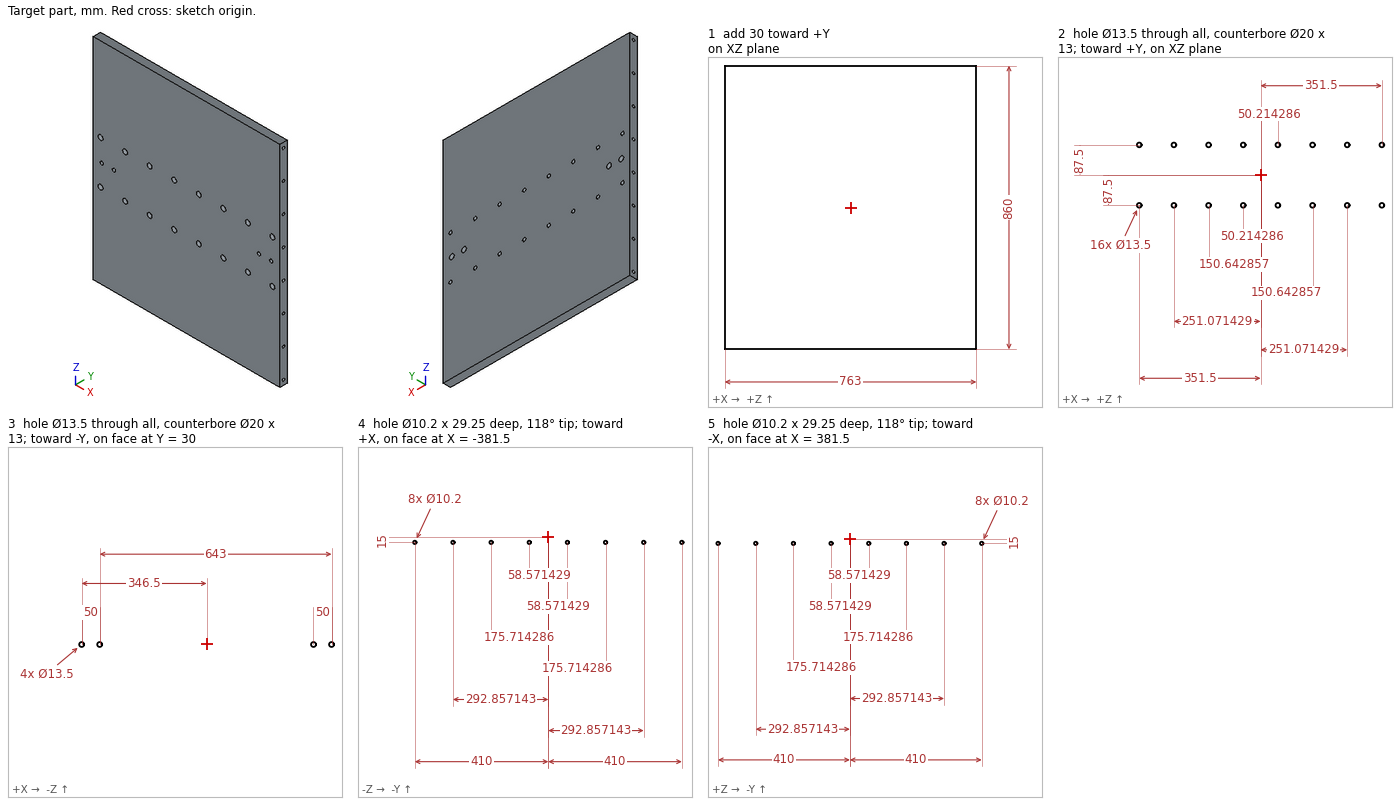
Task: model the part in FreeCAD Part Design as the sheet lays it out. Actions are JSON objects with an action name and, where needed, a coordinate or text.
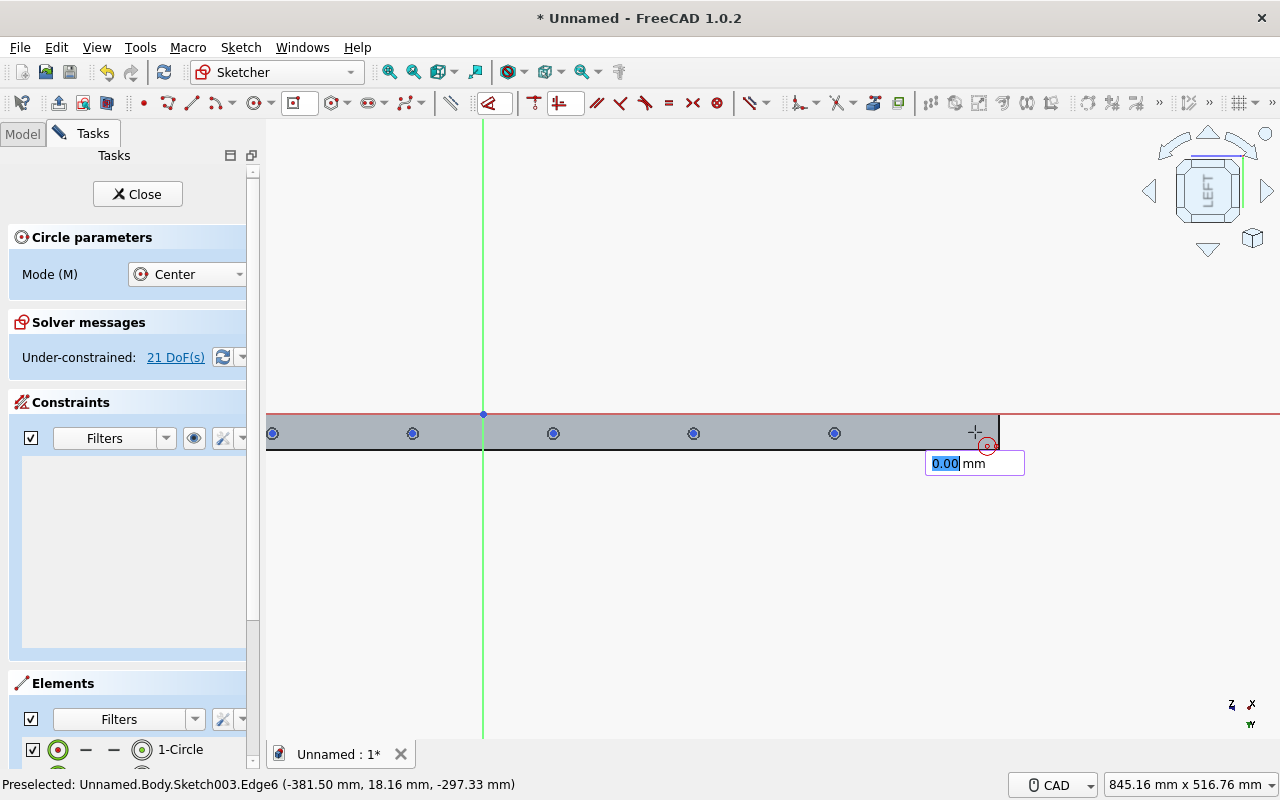
{"action": "scroll", "coordinate": [979, 437], "scroll_direction": "up", "scroll_amount": 5}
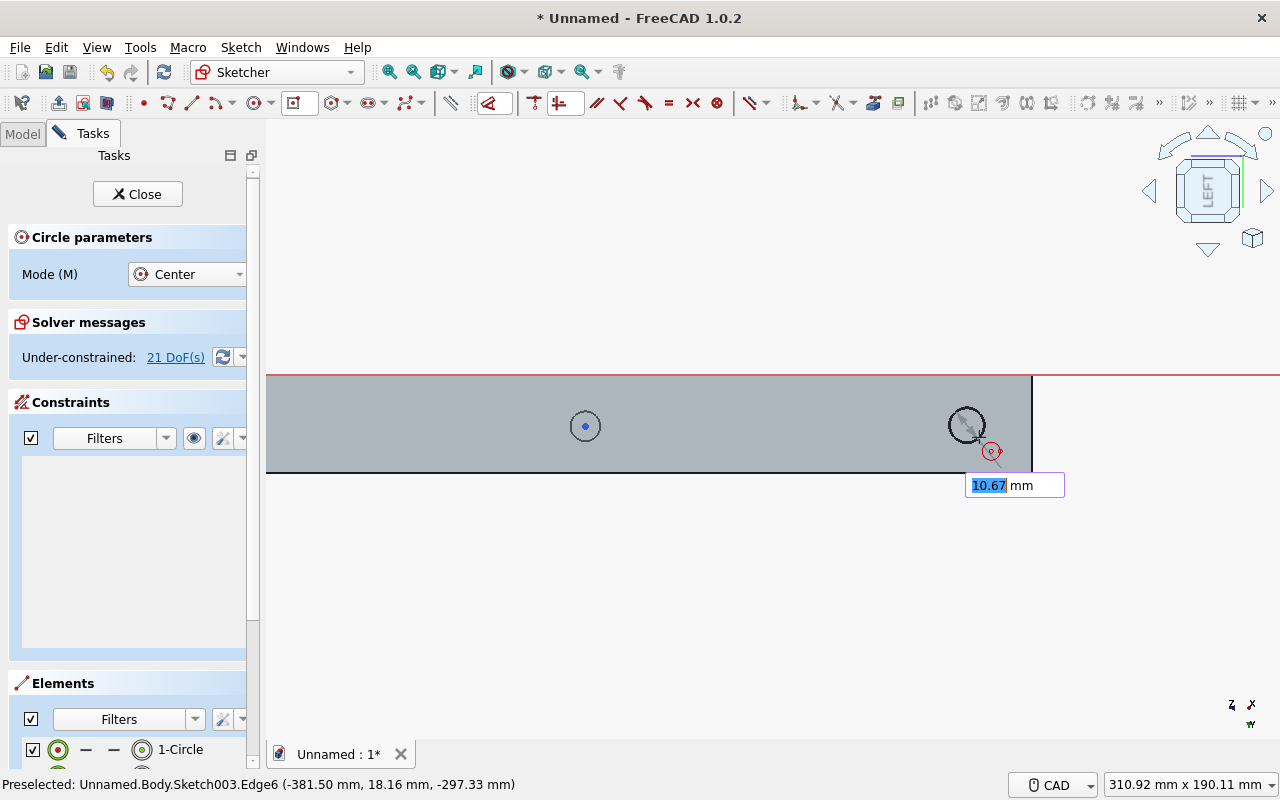
{"action": "left_click", "coordinate": [979, 436]}
{"action": "key", "text": "Escape"}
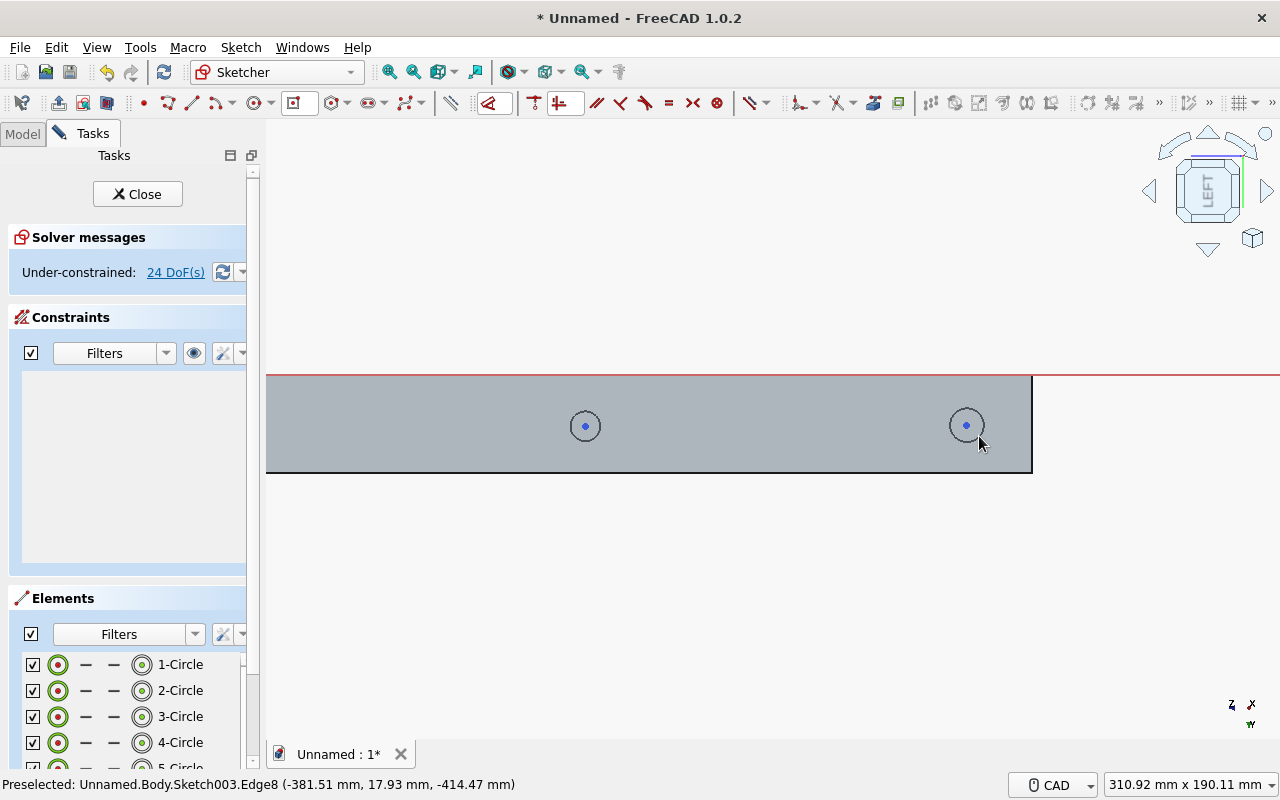
{"action": "scroll", "coordinate": [976, 434], "scroll_direction": "down", "scroll_amount": 8}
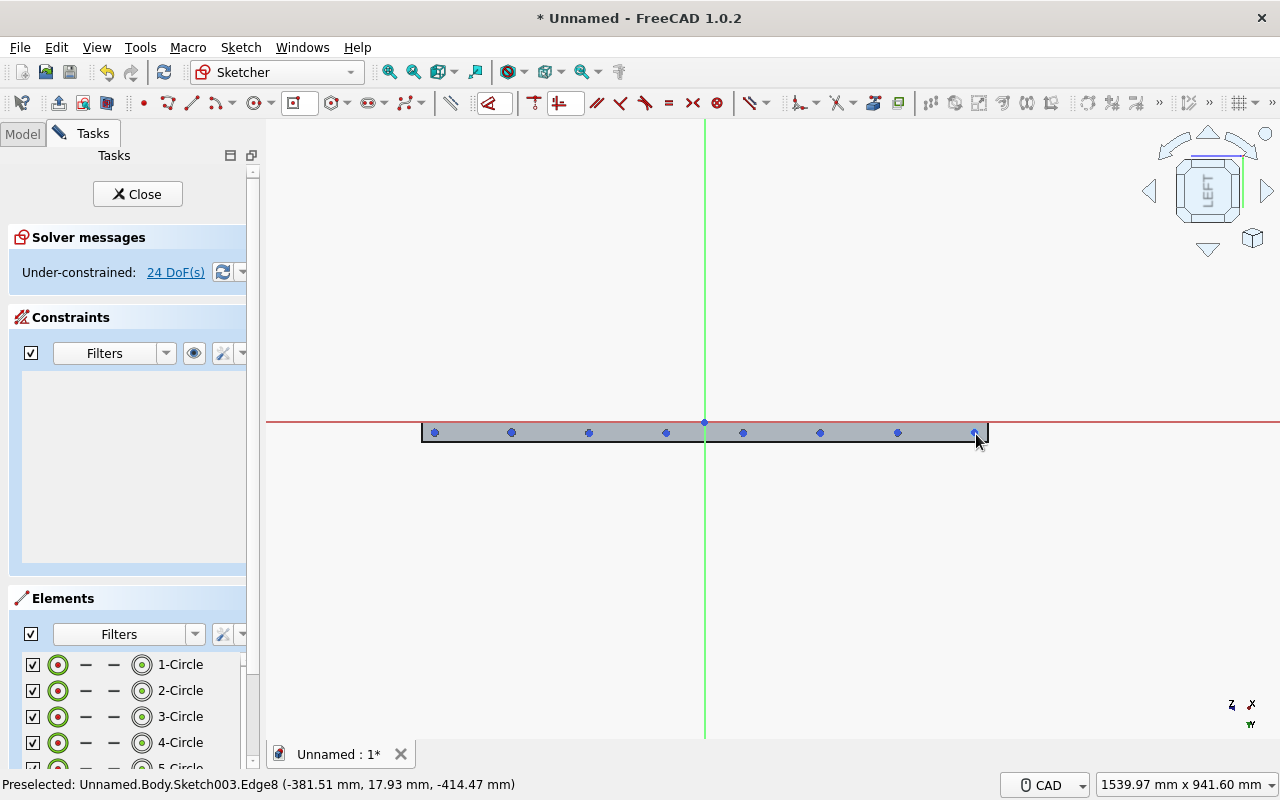
{"action": "scroll", "coordinate": [437, 430], "scroll_direction": "up", "scroll_amount": 8}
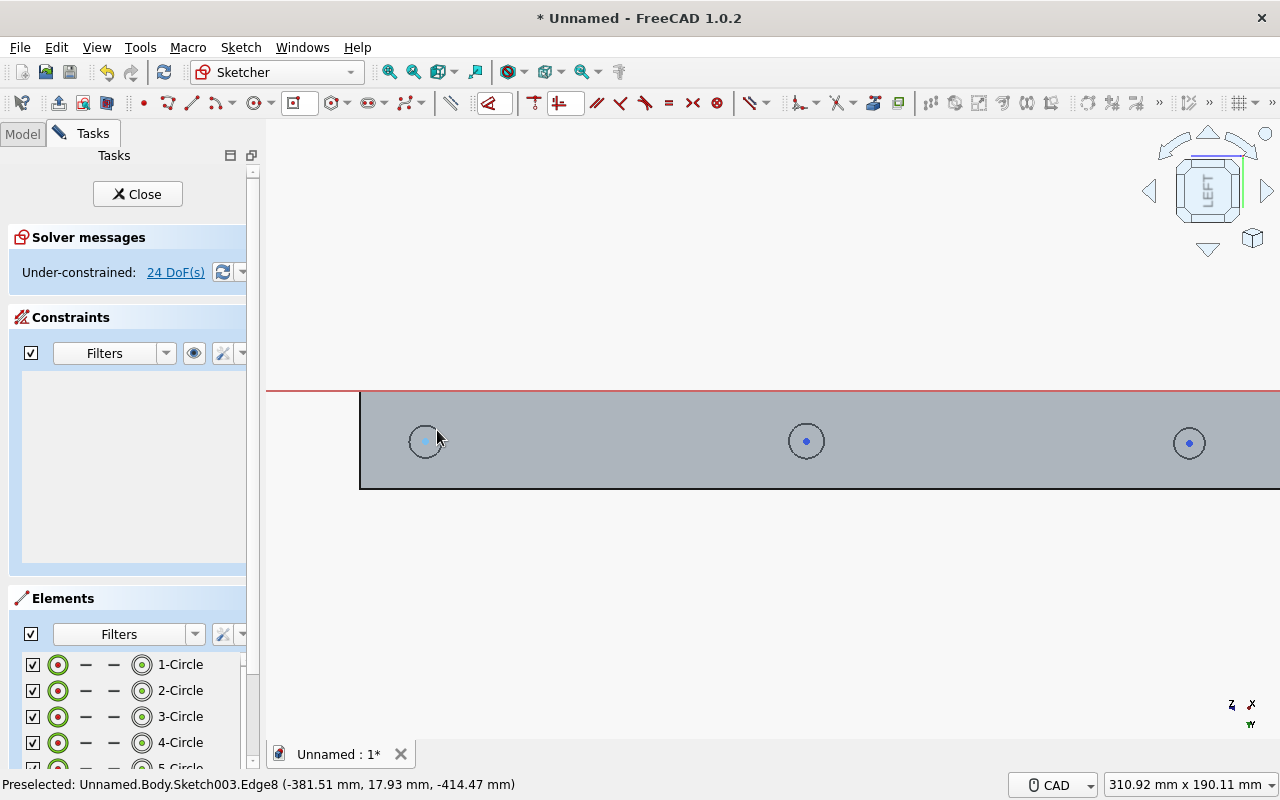
{"action": "left_click", "coordinate": [437, 430]}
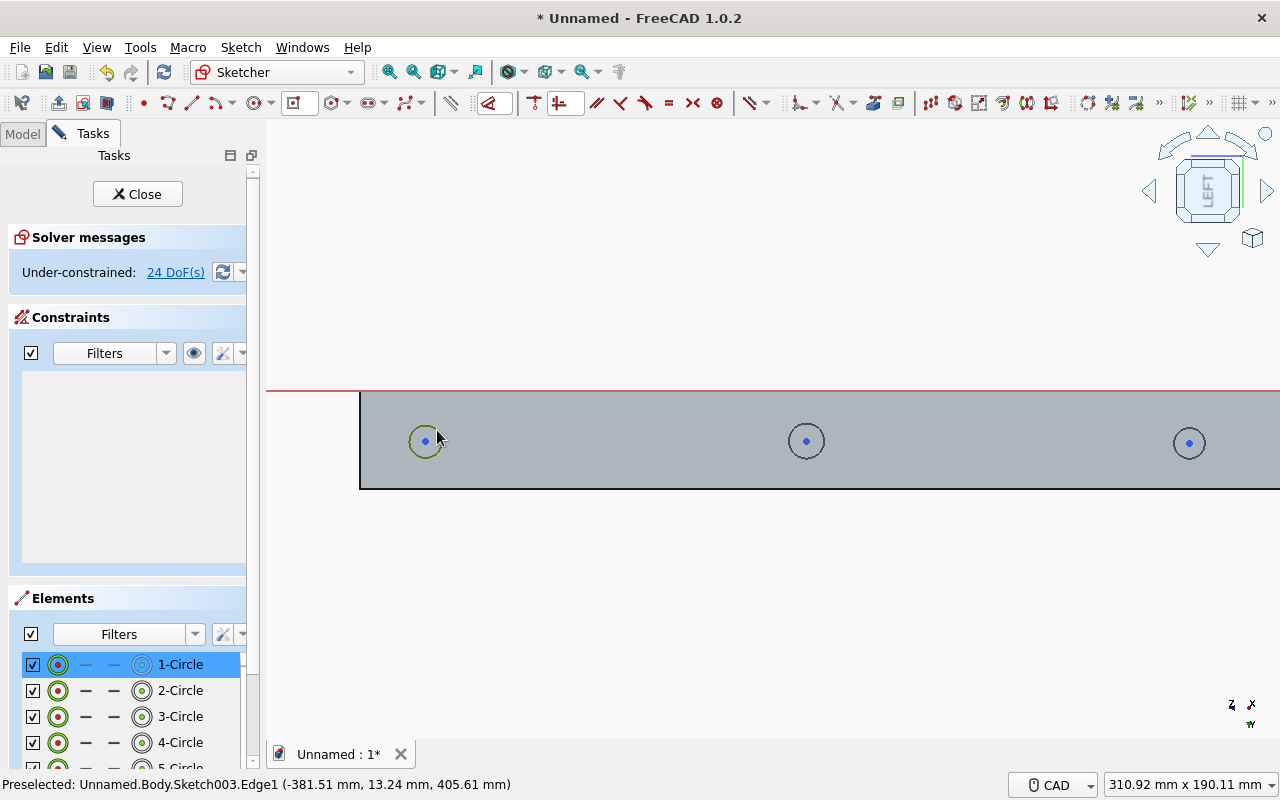
{"action": "left_click", "coordinate": [819, 429]}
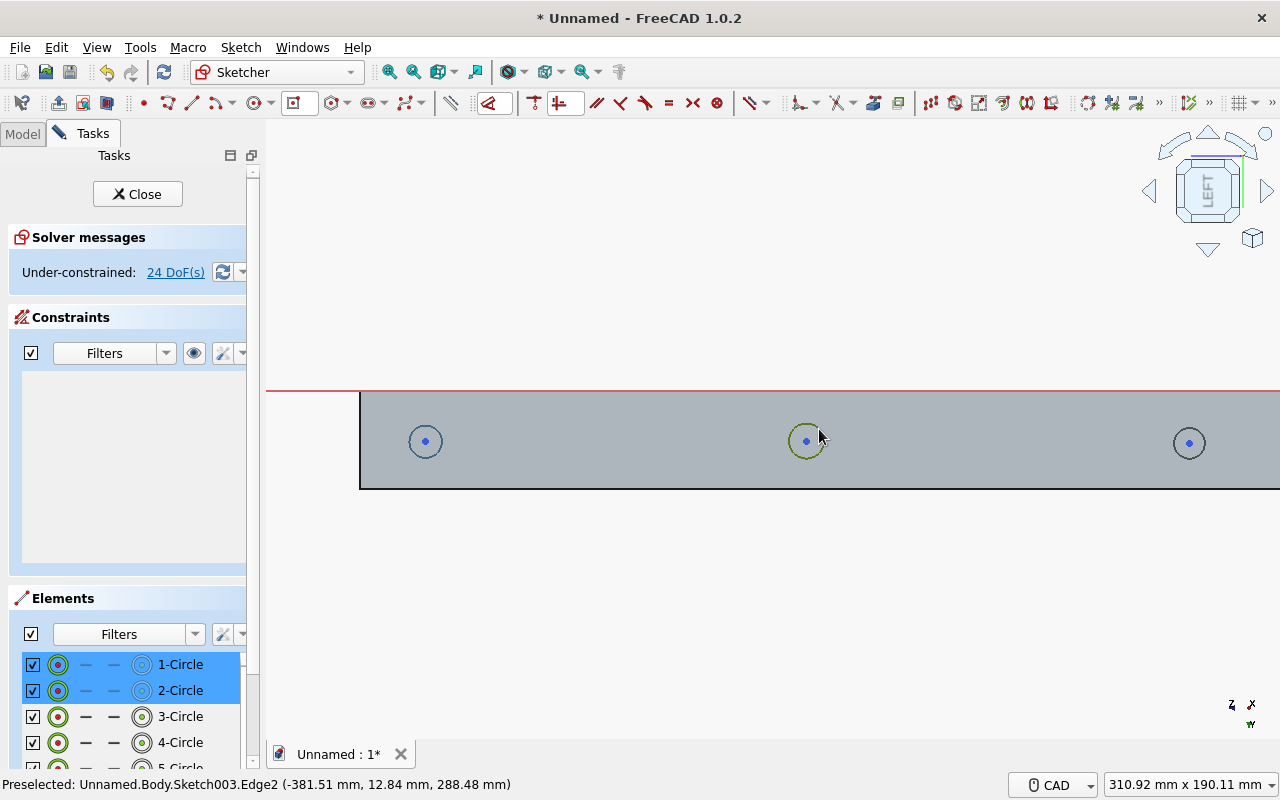
{"action": "scroll", "coordinate": [437, 430], "scroll_direction": "down", "scroll_amount": 8}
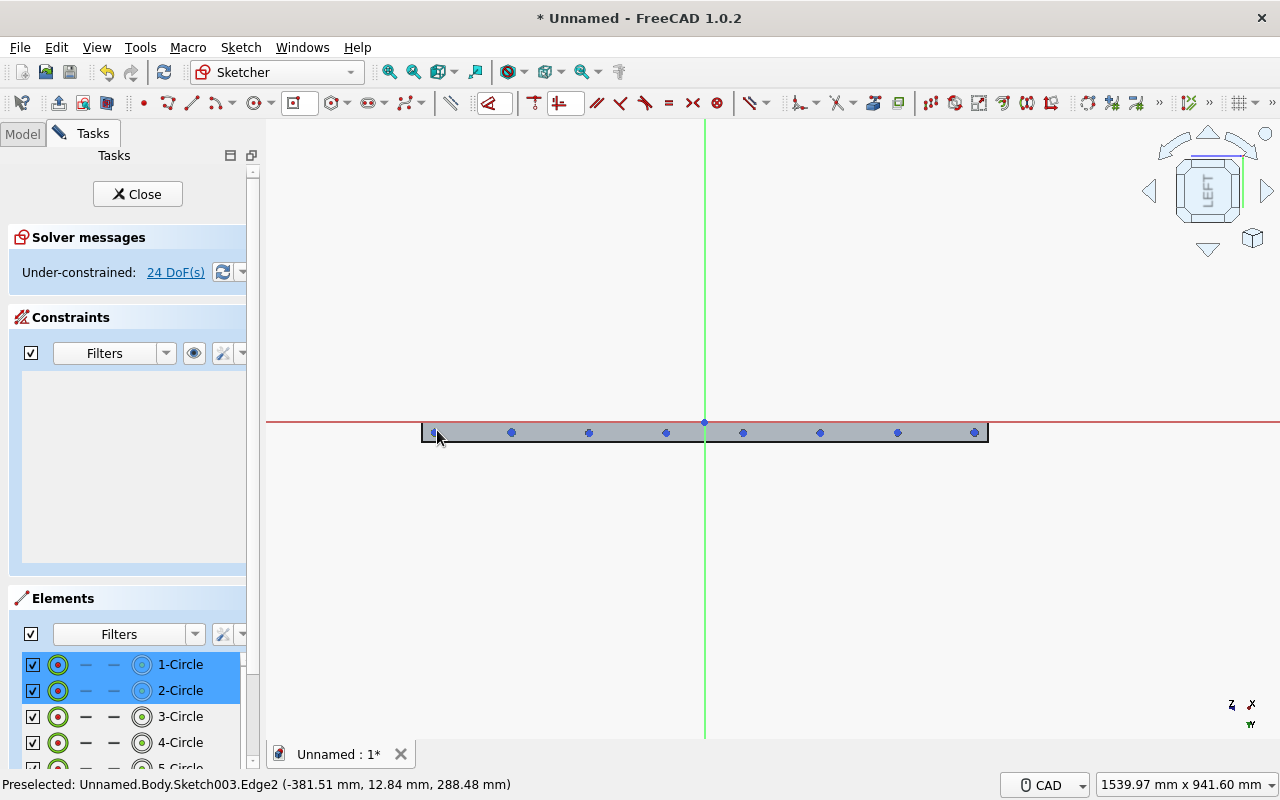
{"action": "scroll", "coordinate": [591, 431], "scroll_direction": "up", "scroll_amount": 8}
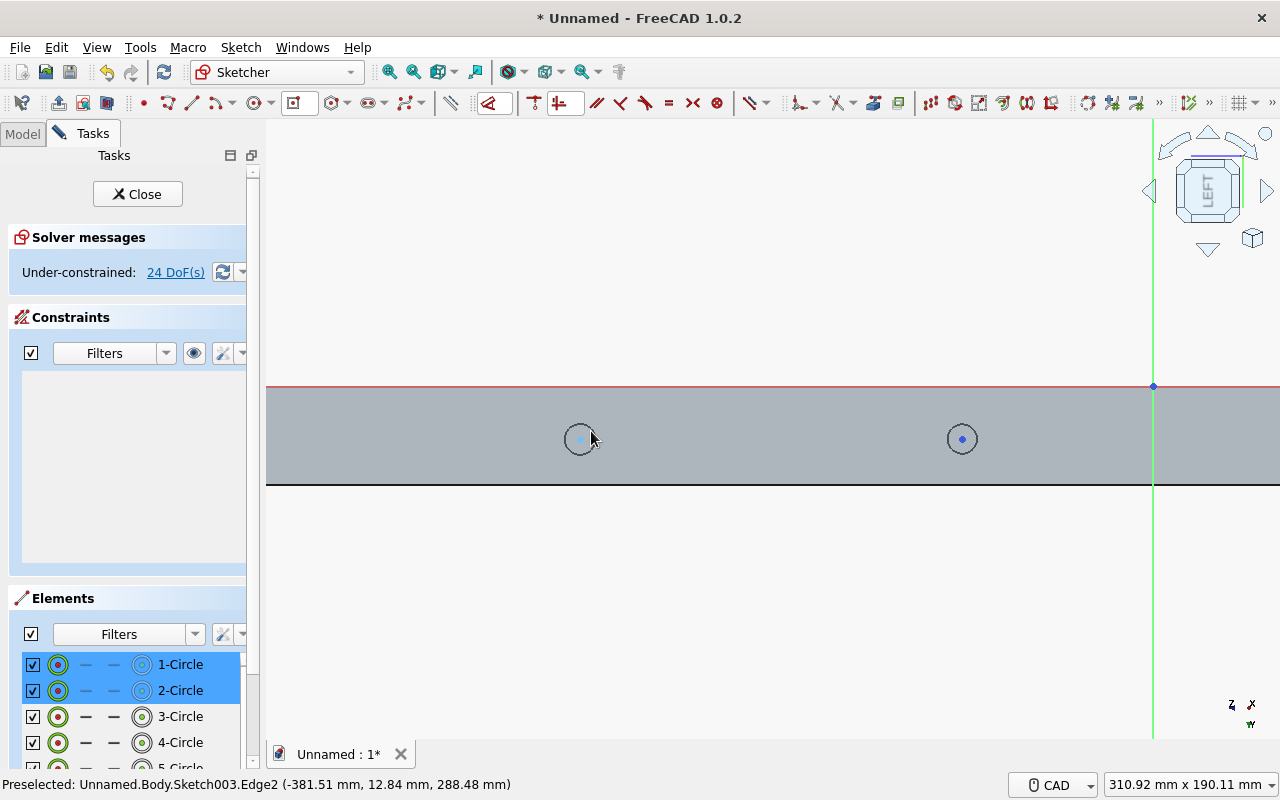
{"action": "left_click", "coordinate": [591, 429]}